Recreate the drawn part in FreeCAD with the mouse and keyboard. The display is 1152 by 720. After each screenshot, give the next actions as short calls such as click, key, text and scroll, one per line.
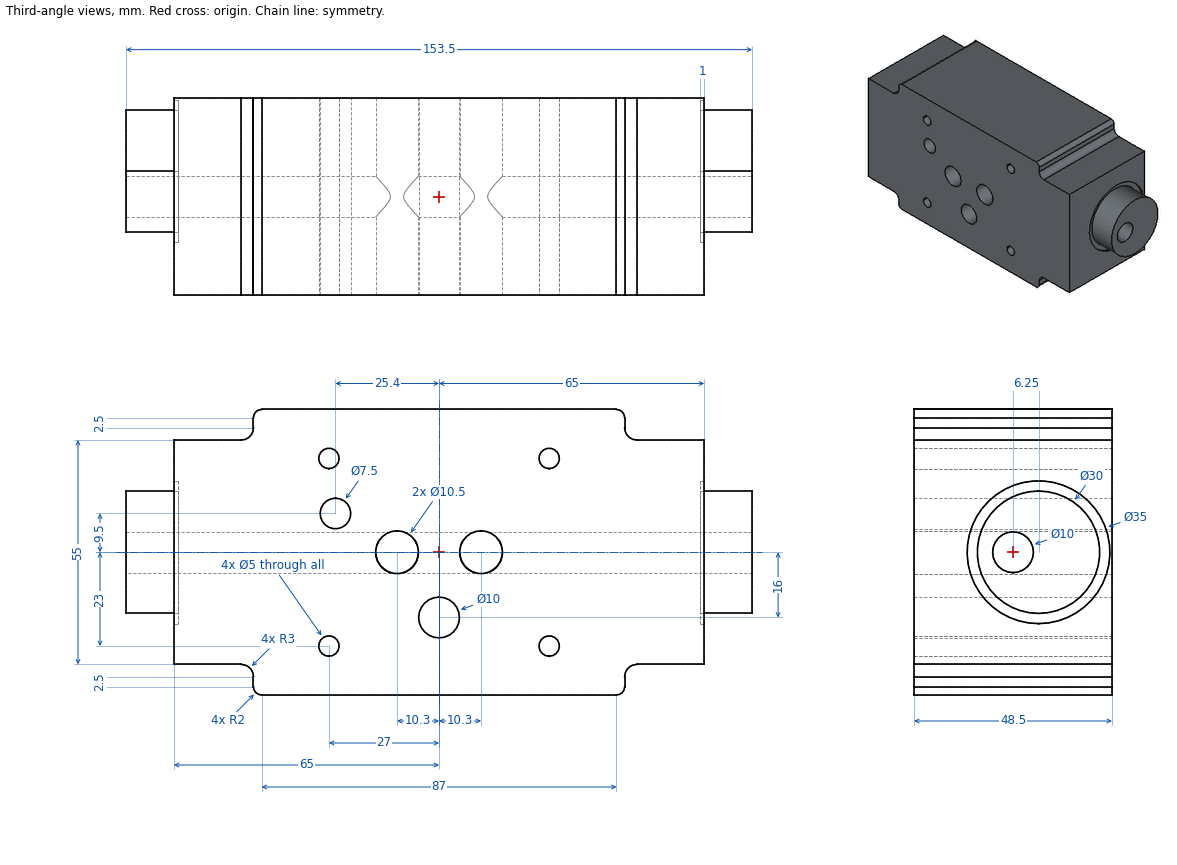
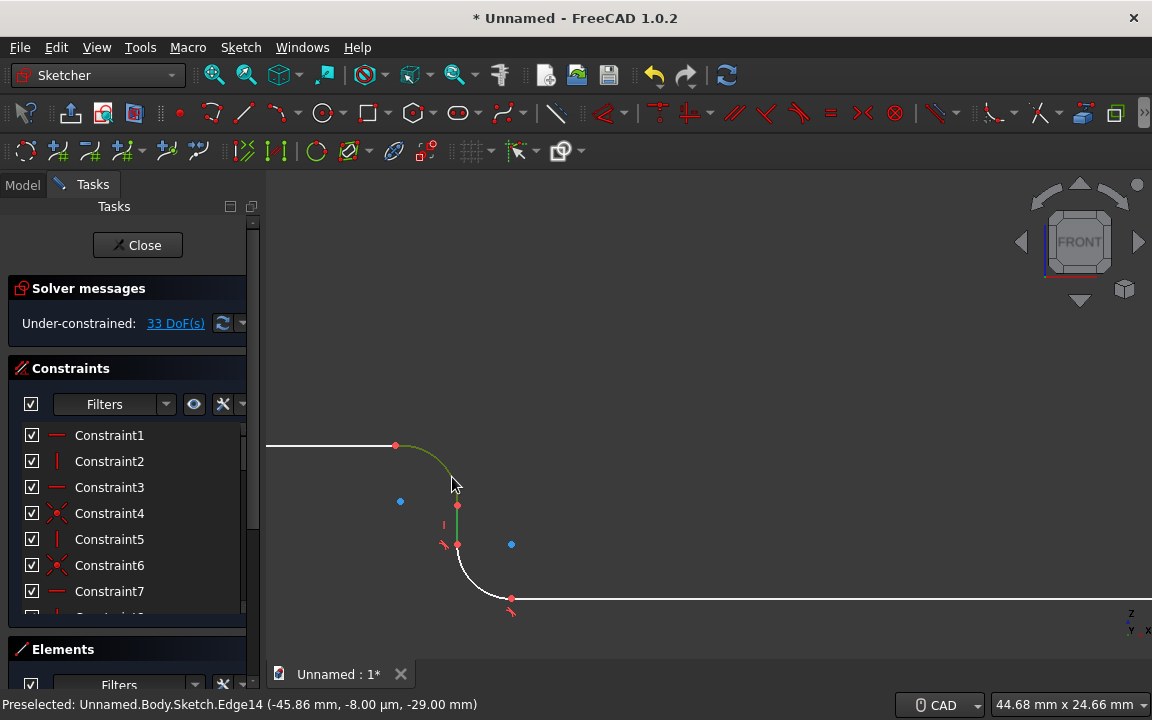
click(800, 114)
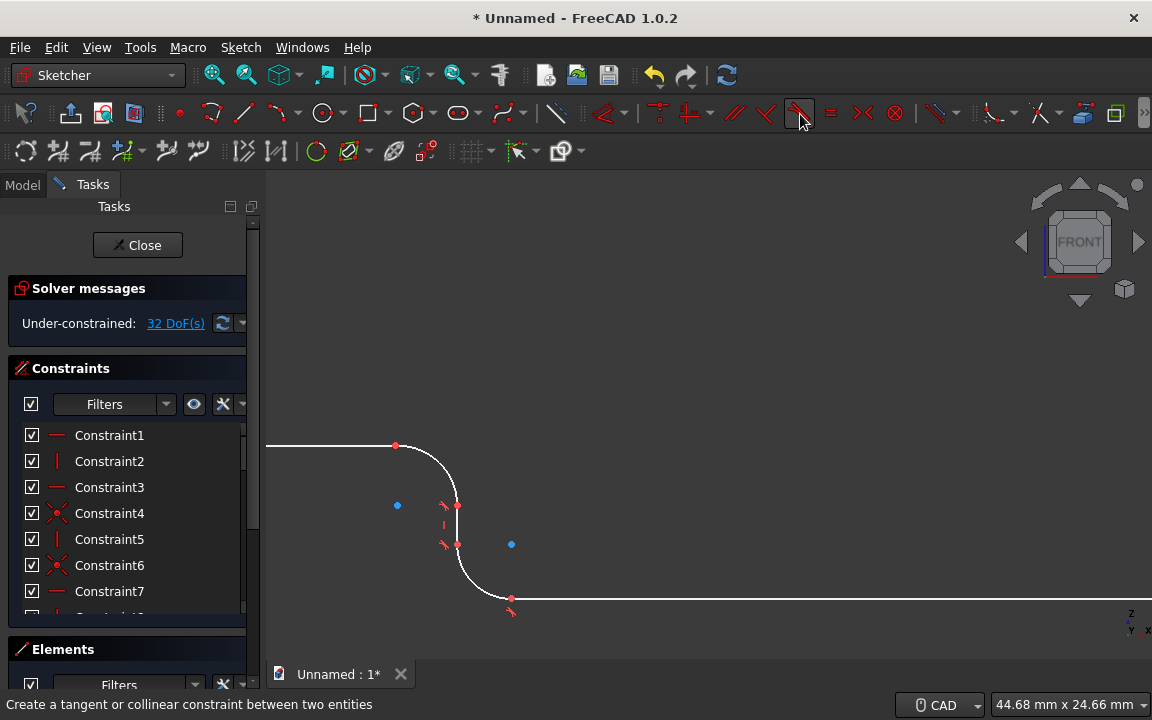
scroll(459, 545, down, 8)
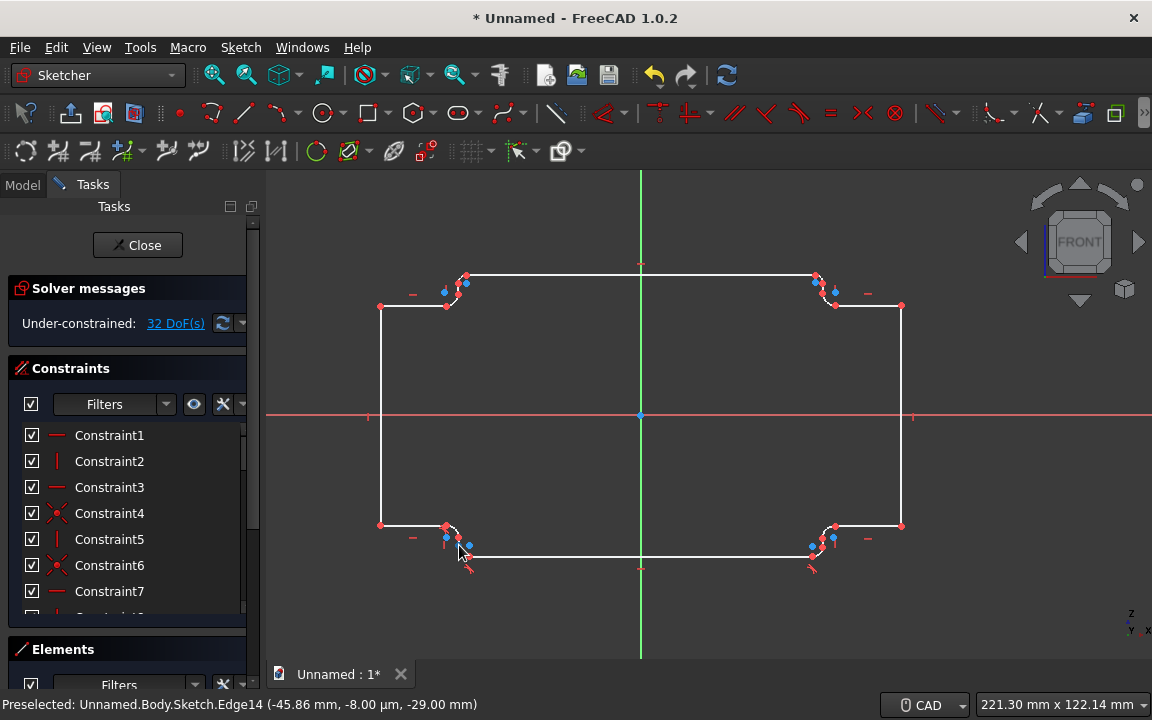
click(427, 526)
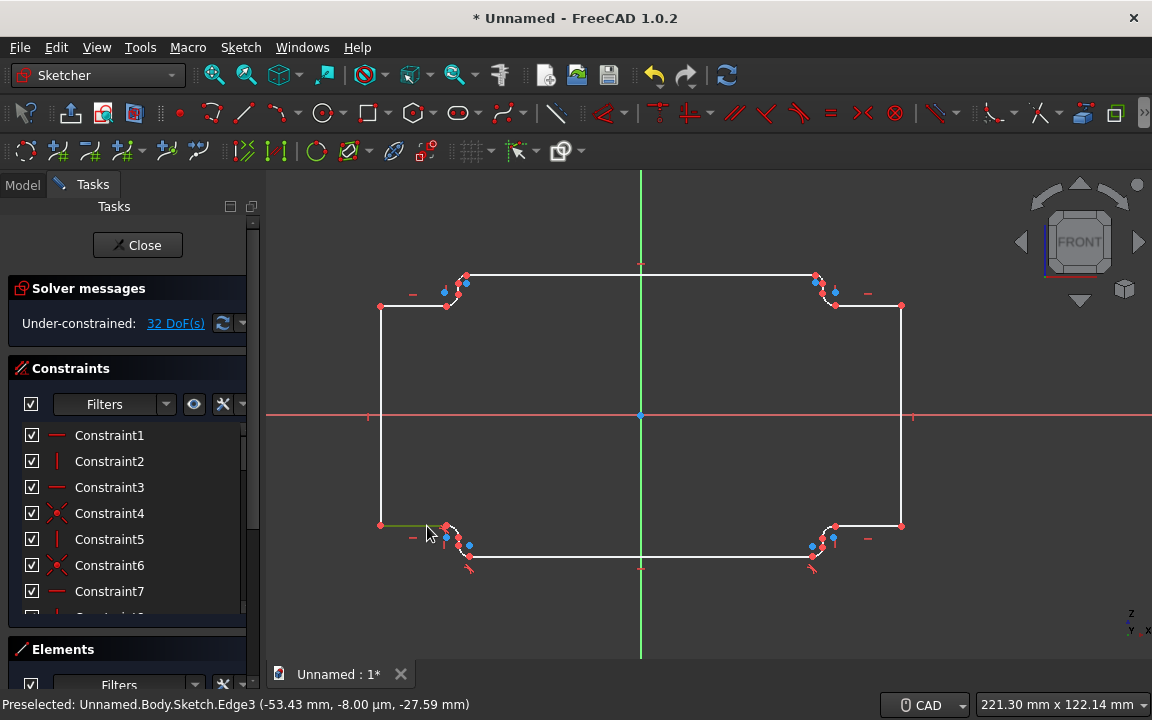
scroll(455, 529, up, 2)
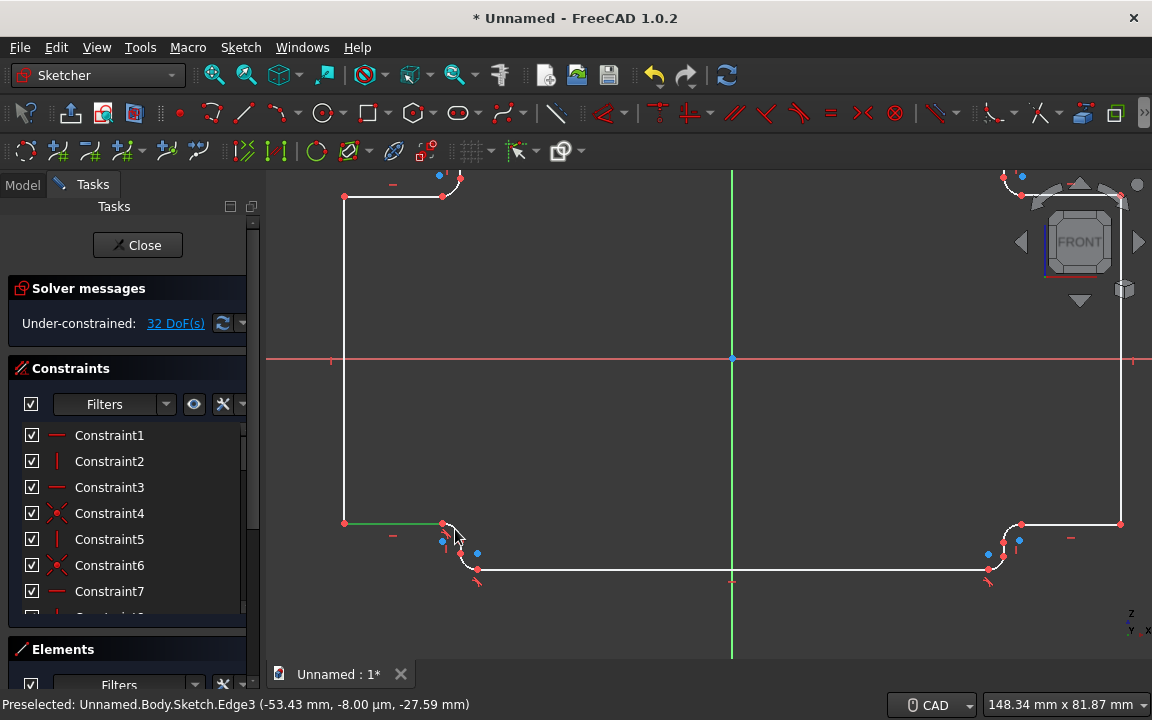
click(450, 525)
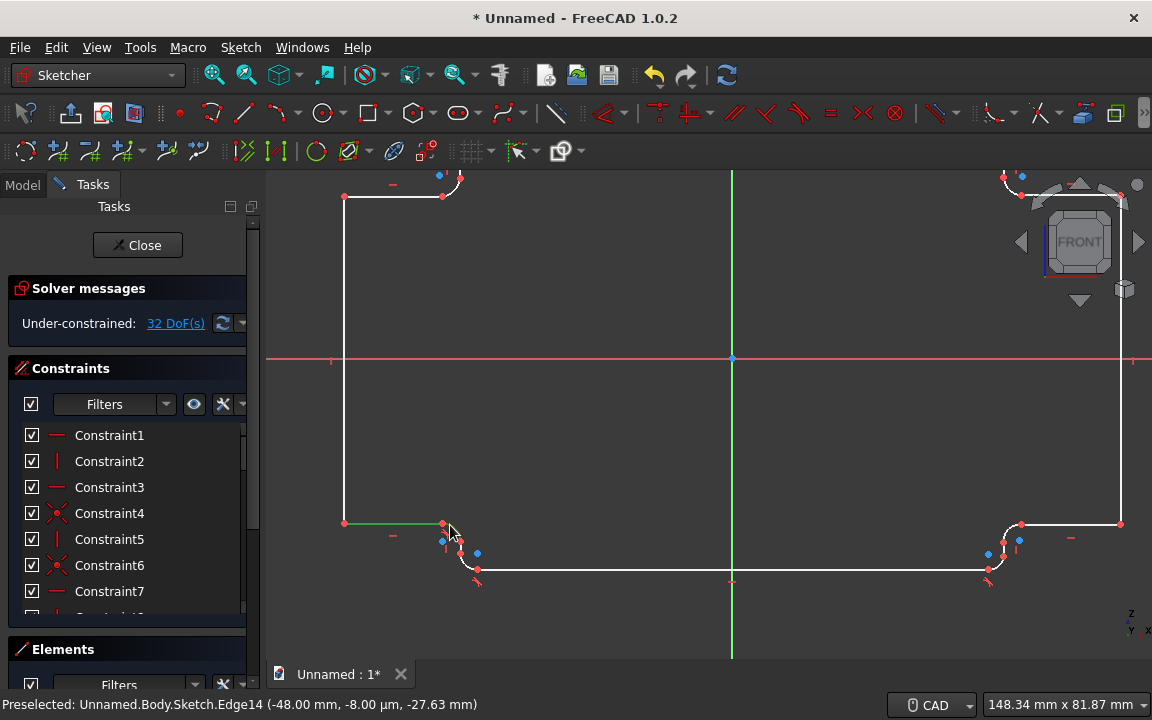
click(800, 114)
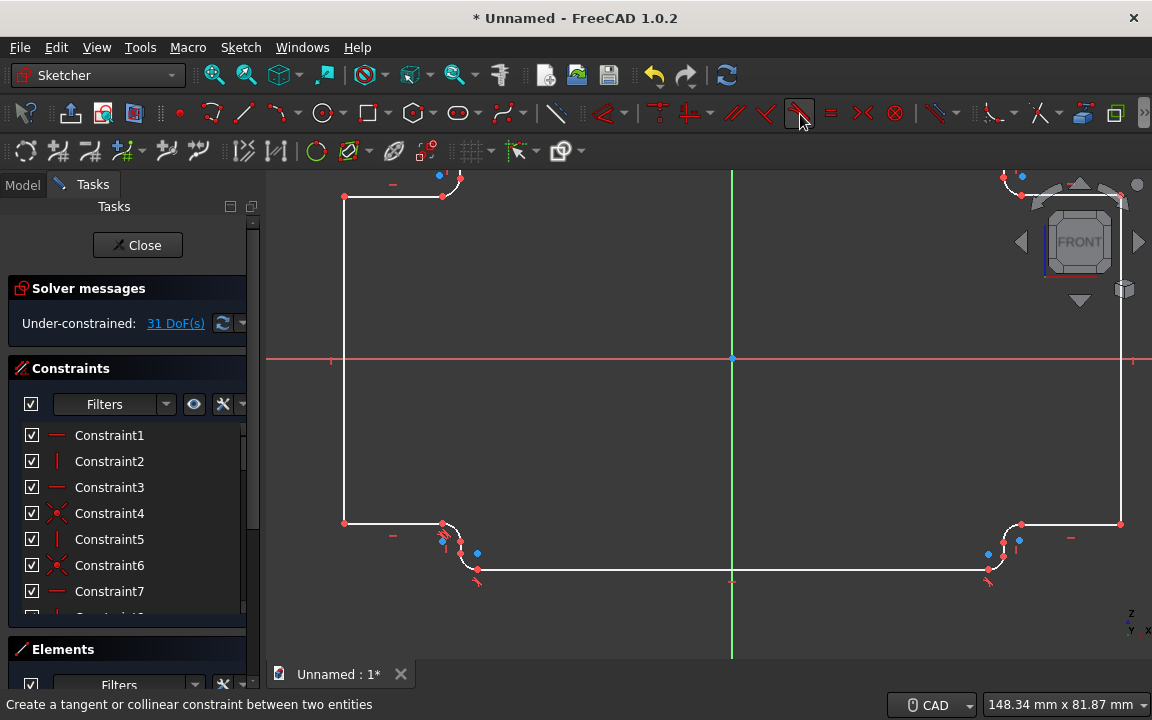
scroll(454, 528, down, 2)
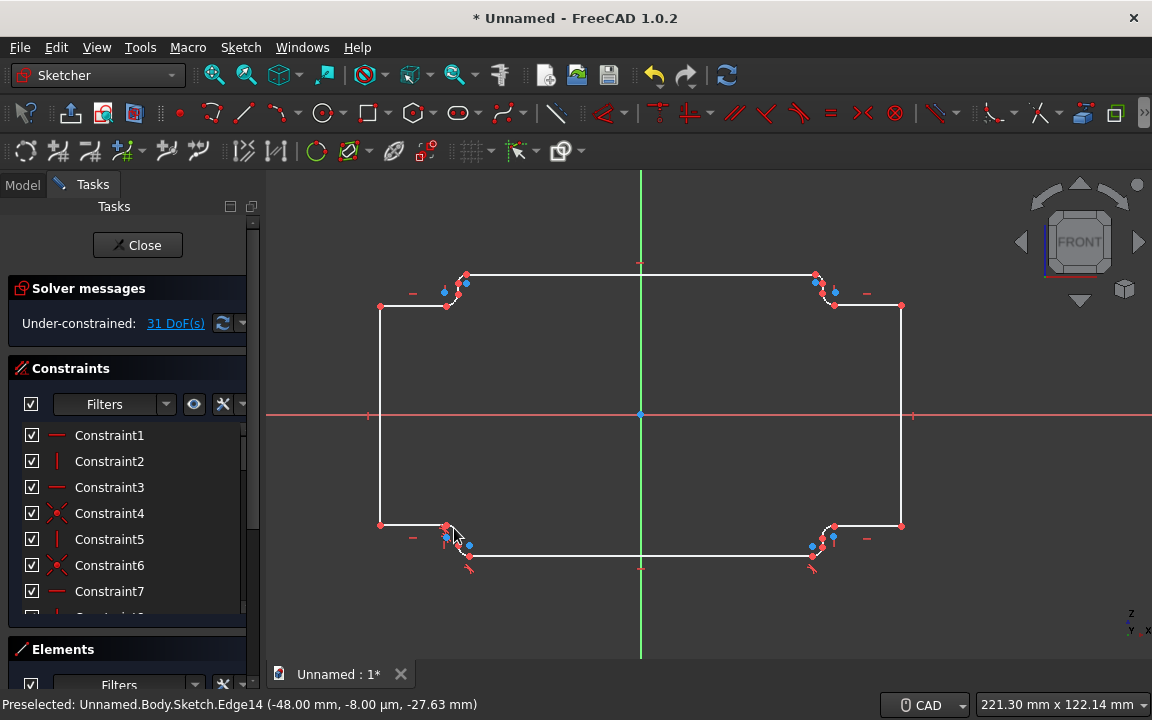
click(400, 306)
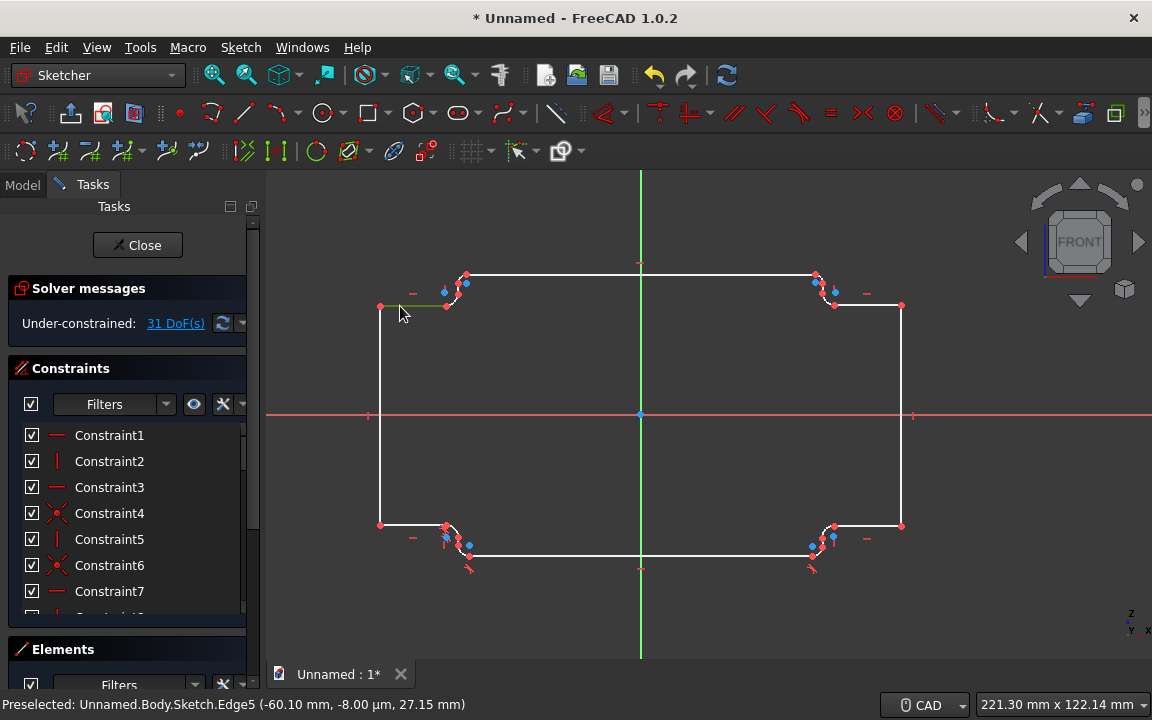
scroll(454, 302, up, 3)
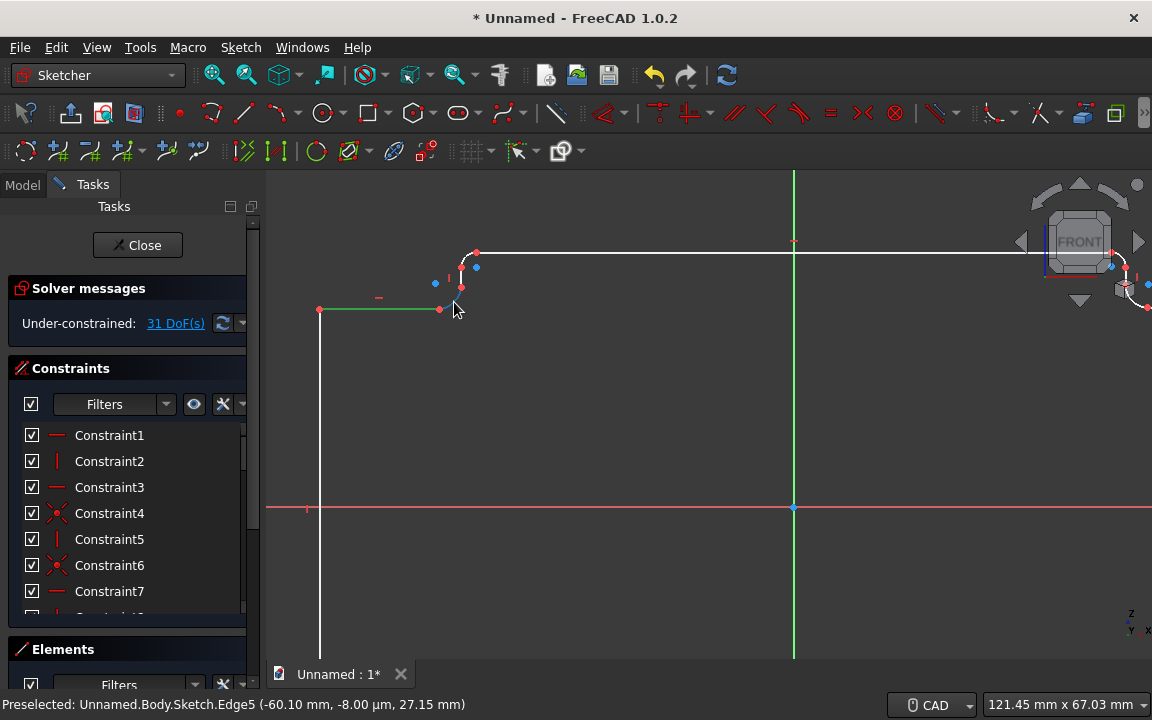
click(454, 302)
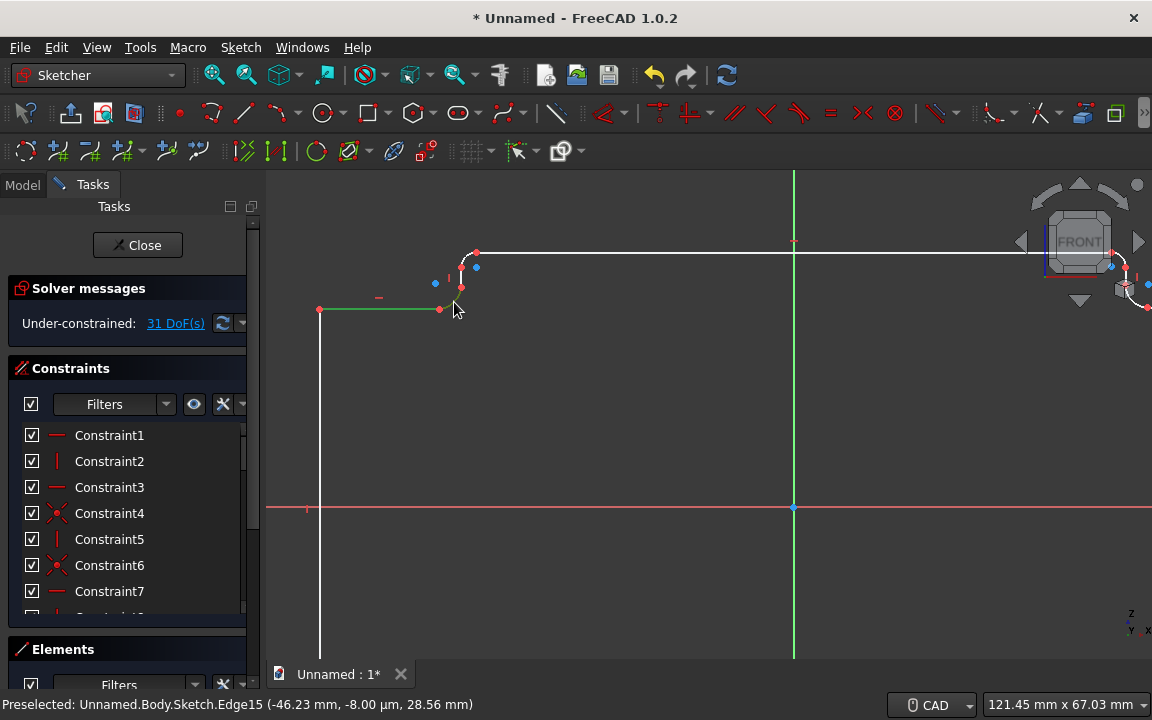
click(800, 114)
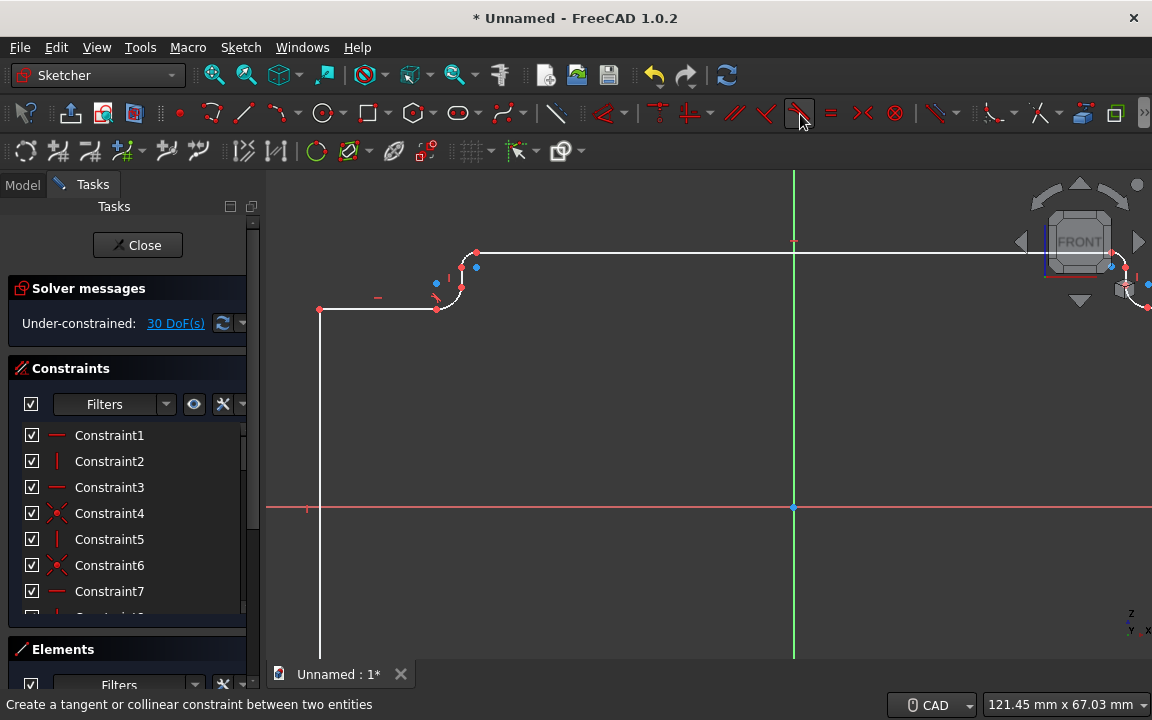
scroll(462, 277, up, 2)